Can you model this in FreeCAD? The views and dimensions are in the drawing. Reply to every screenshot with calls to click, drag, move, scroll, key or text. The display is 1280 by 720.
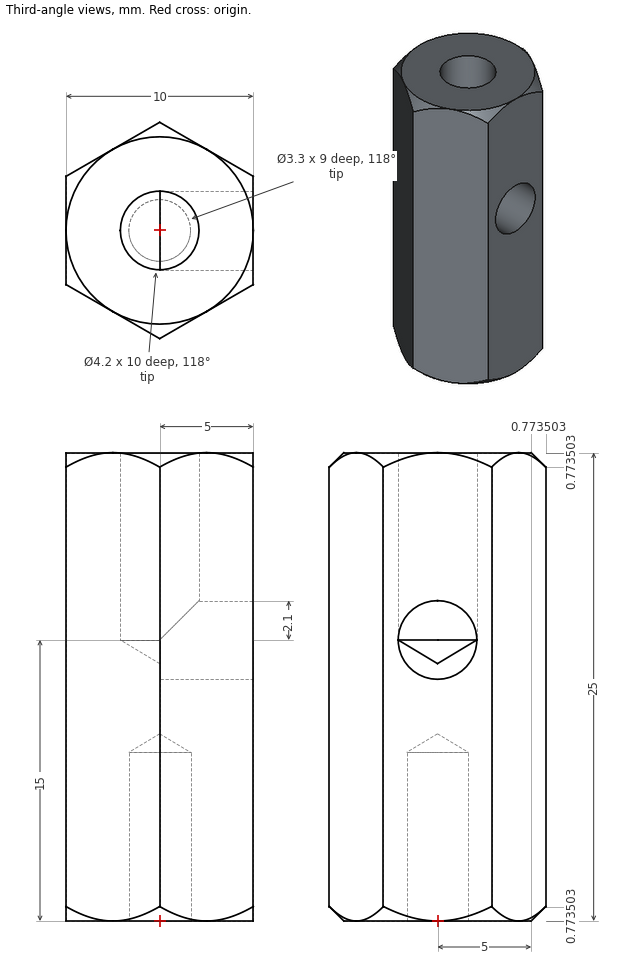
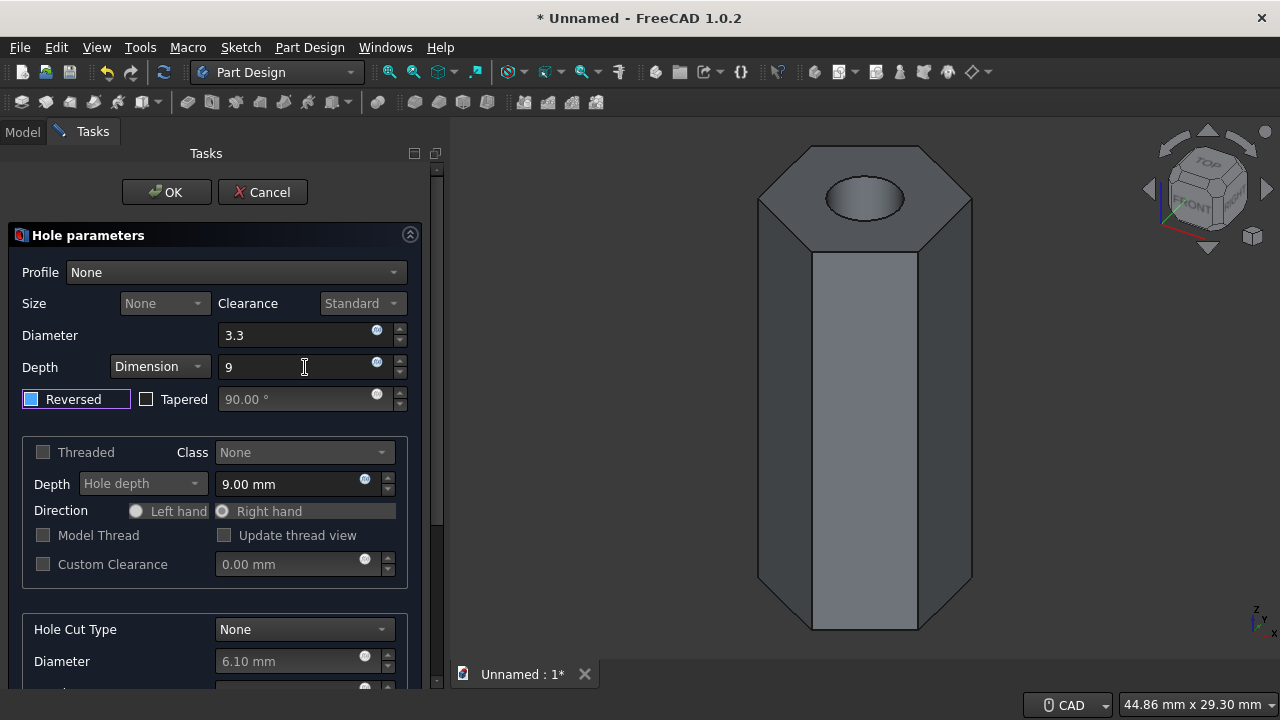
click(30, 399)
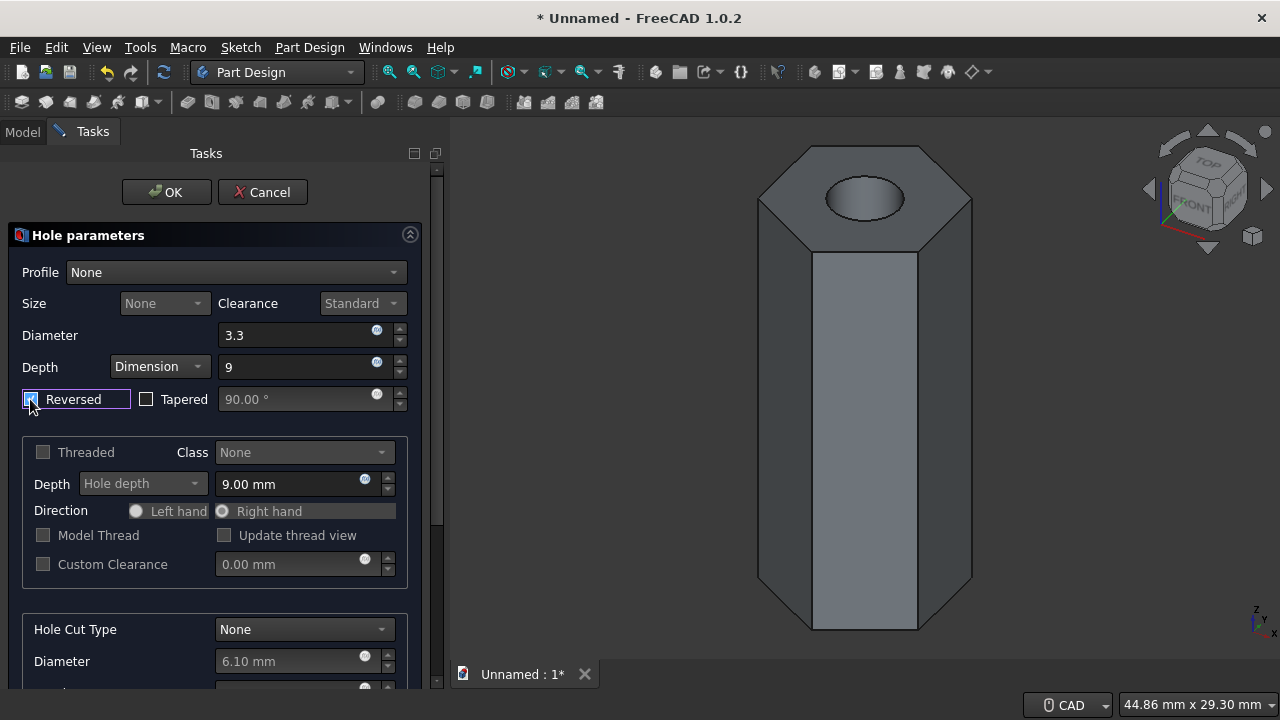
click(167, 192)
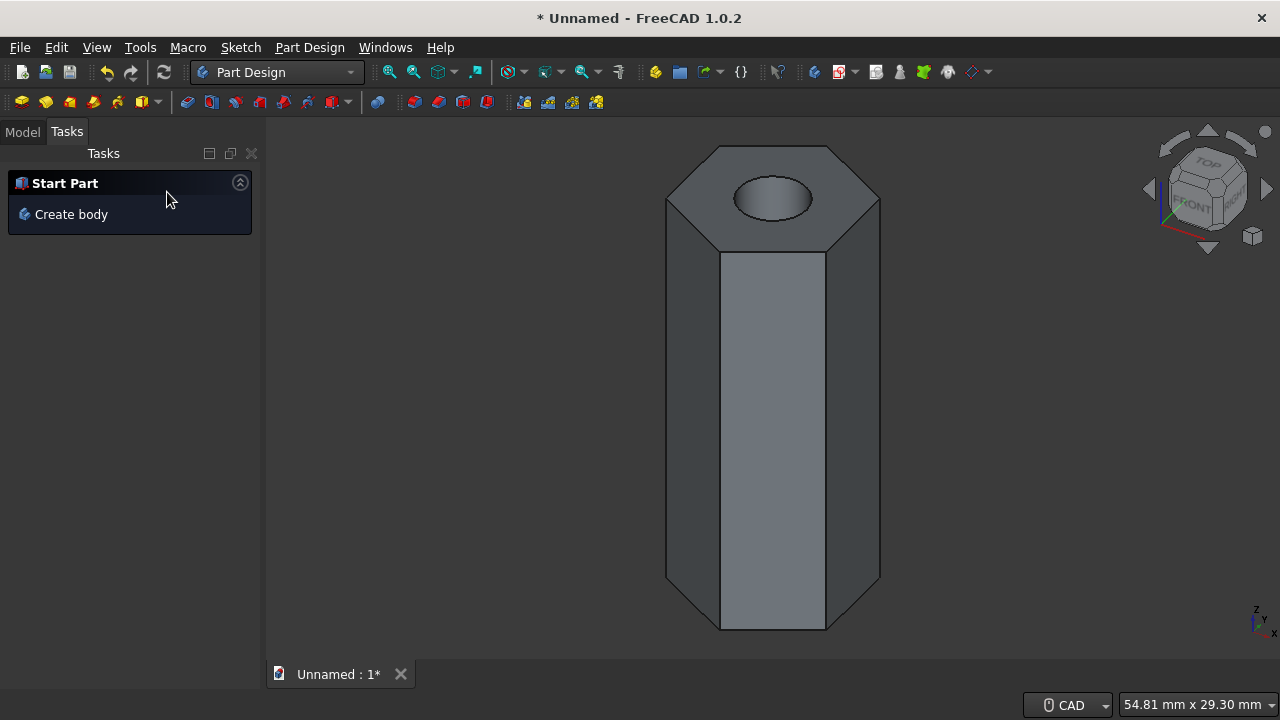
click(840, 72)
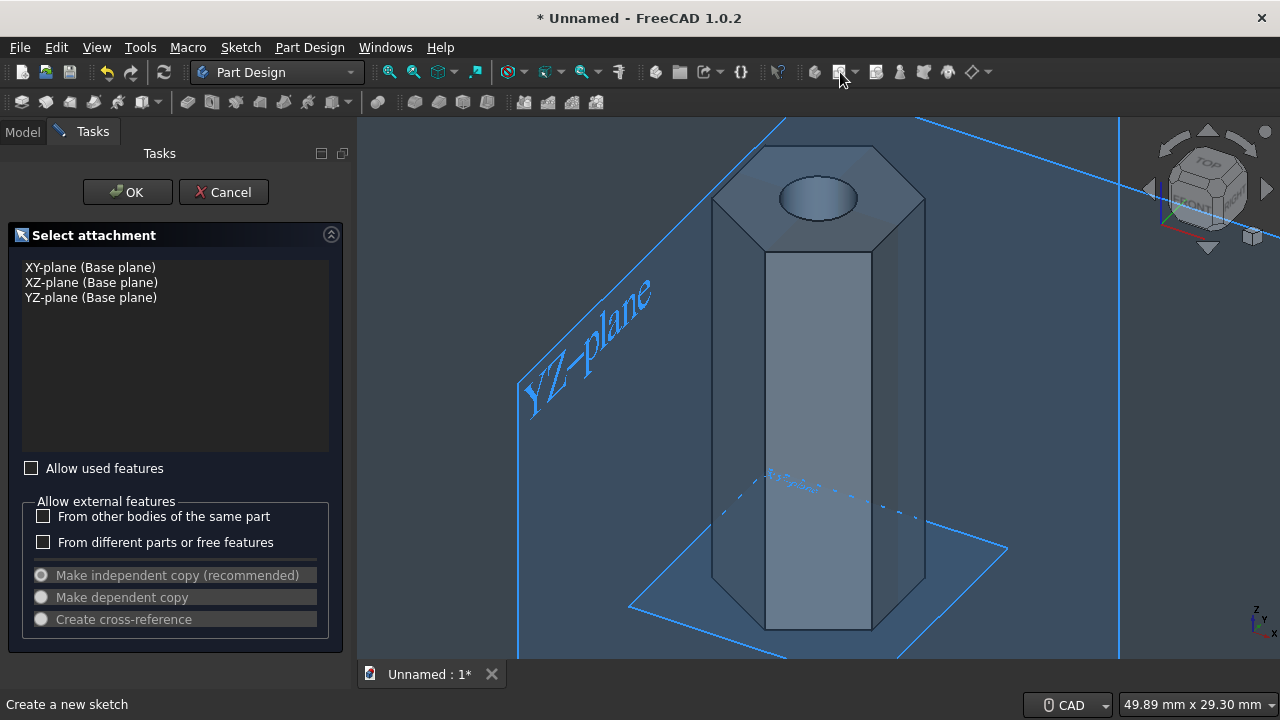
click(82, 282)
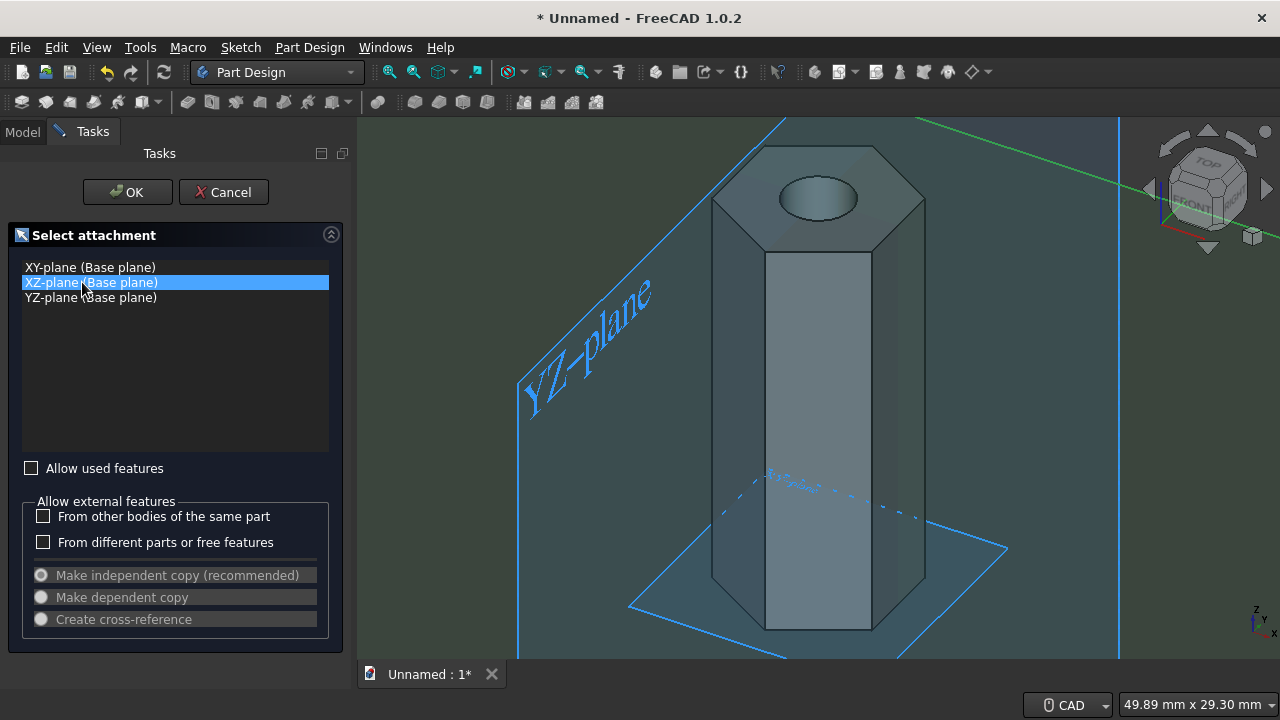
click(128, 192)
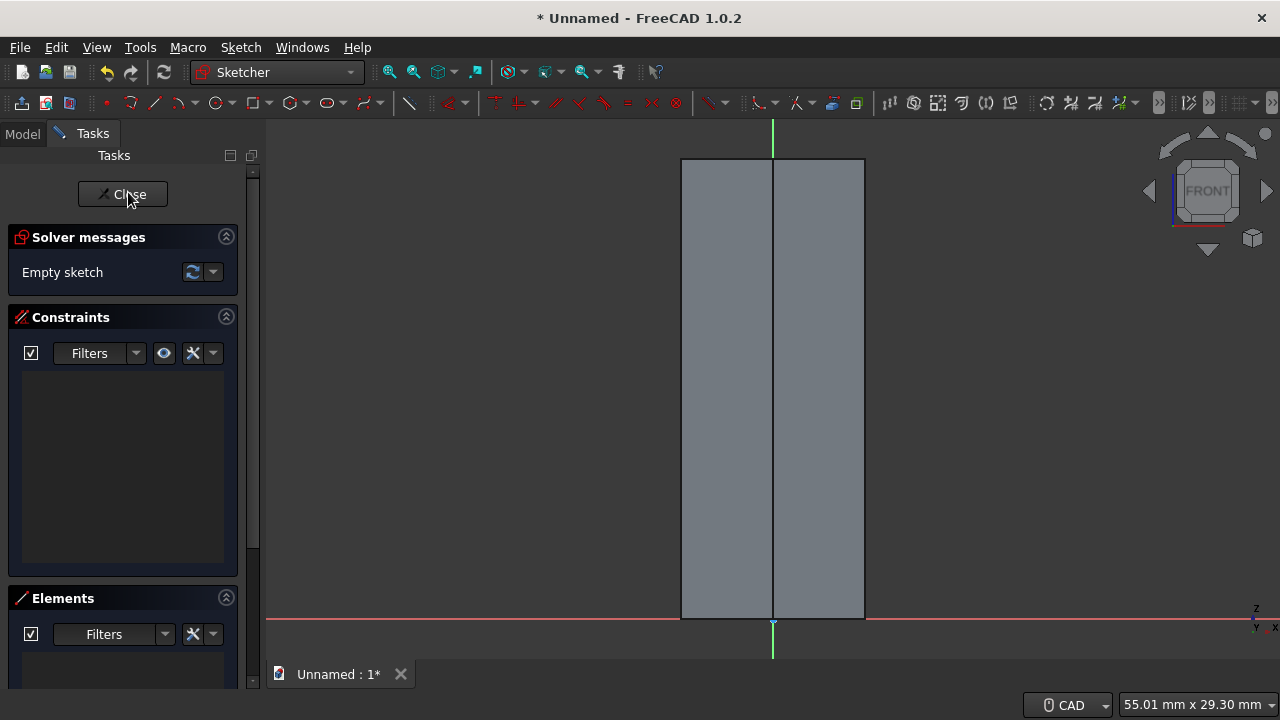
key(q)
key(s)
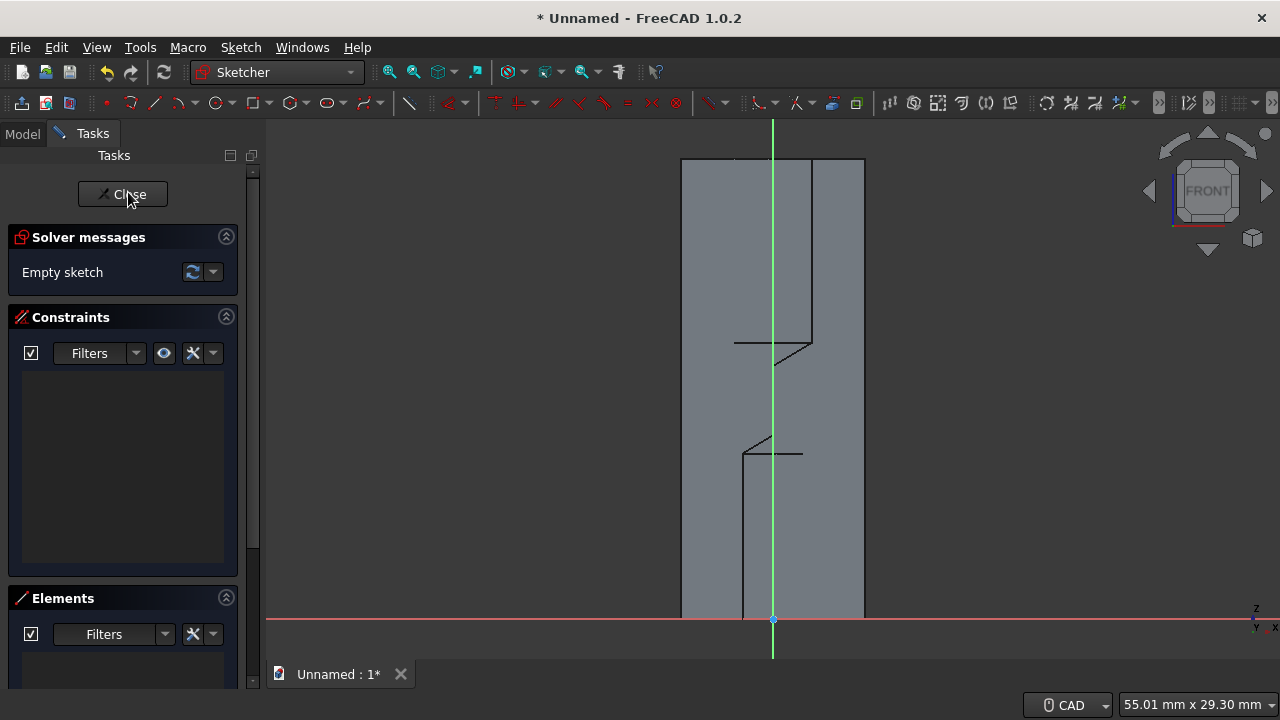
scroll(294, 147, down, 1)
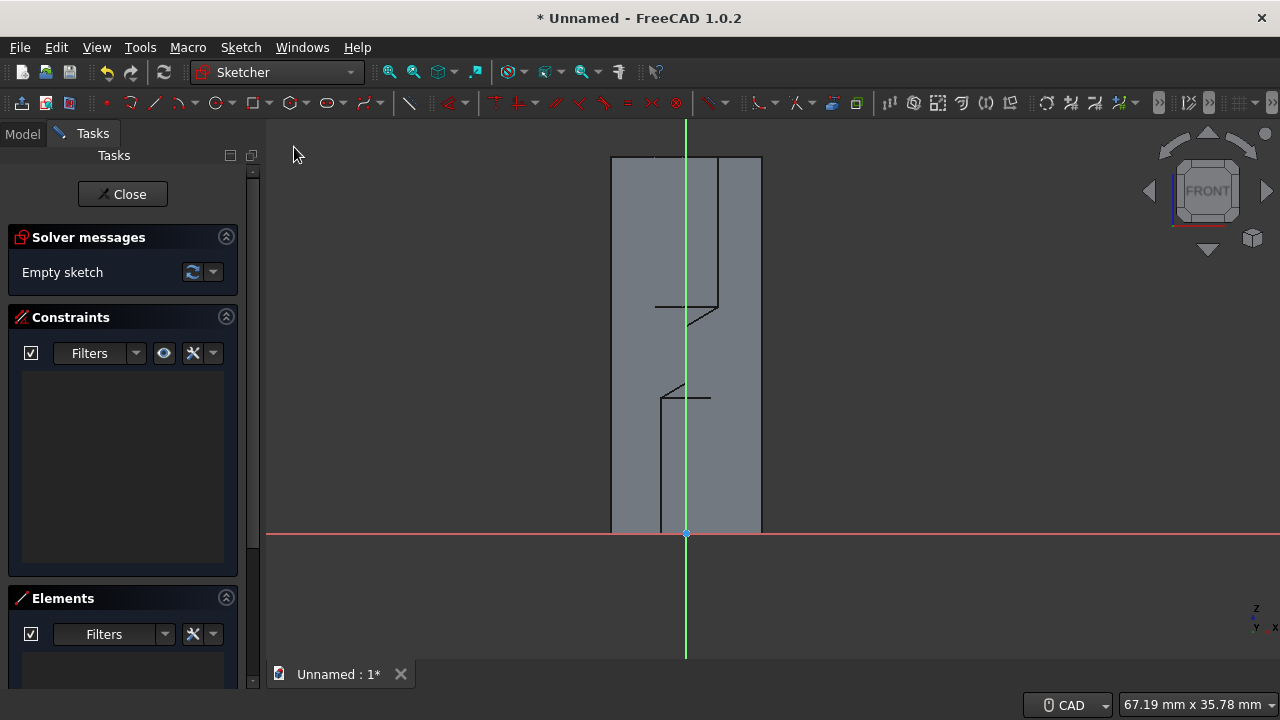
key(g)
key(r)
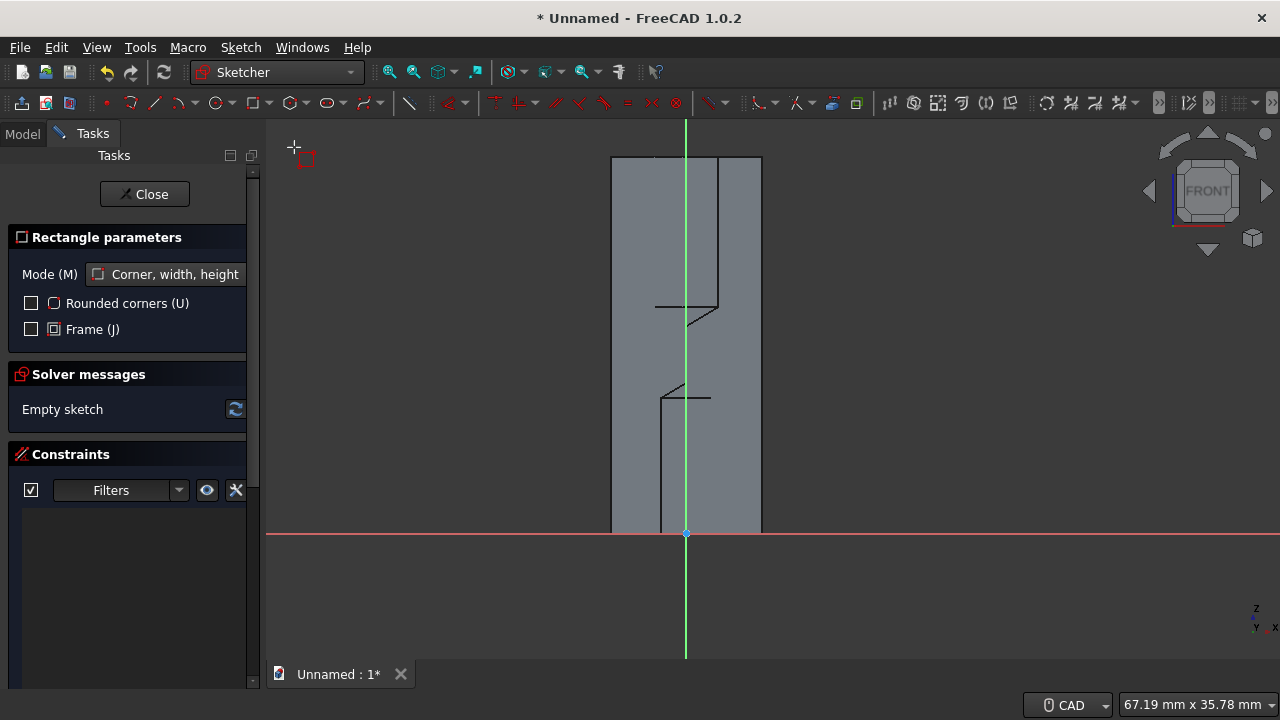
click(686, 276)
move(762, 307)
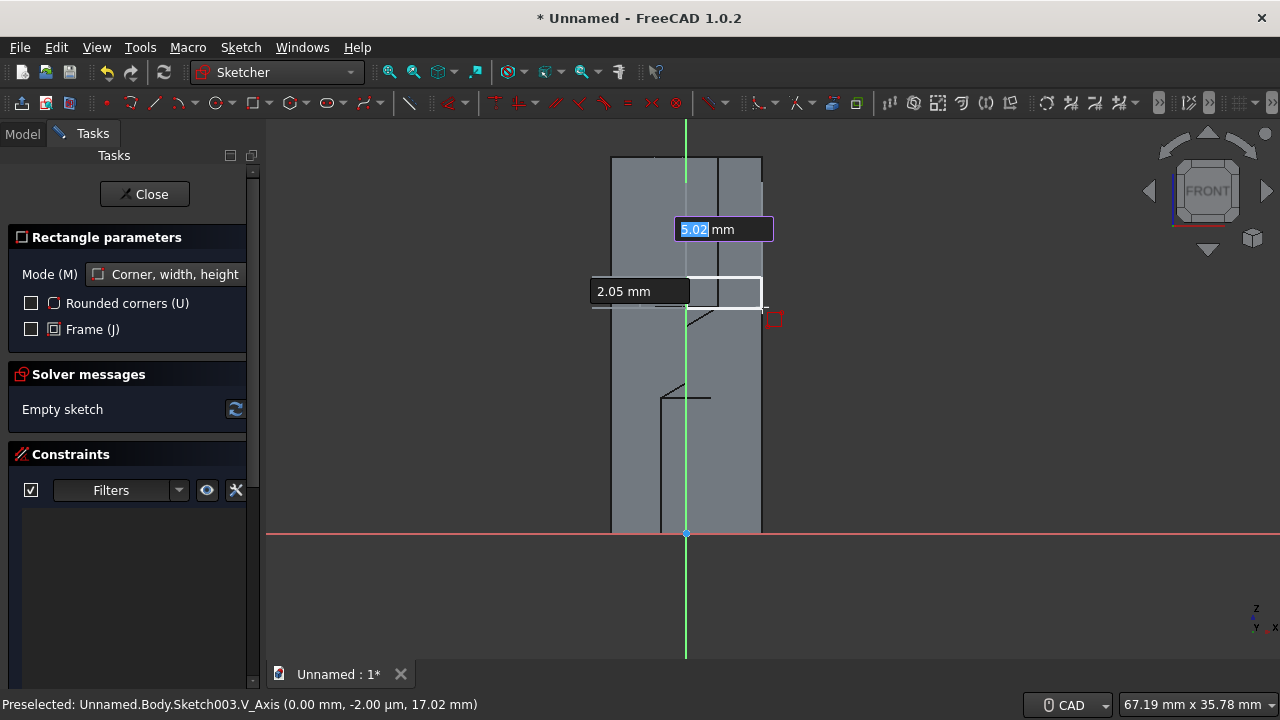
text(5)
key(Tab)
text(2.1)
key(Return)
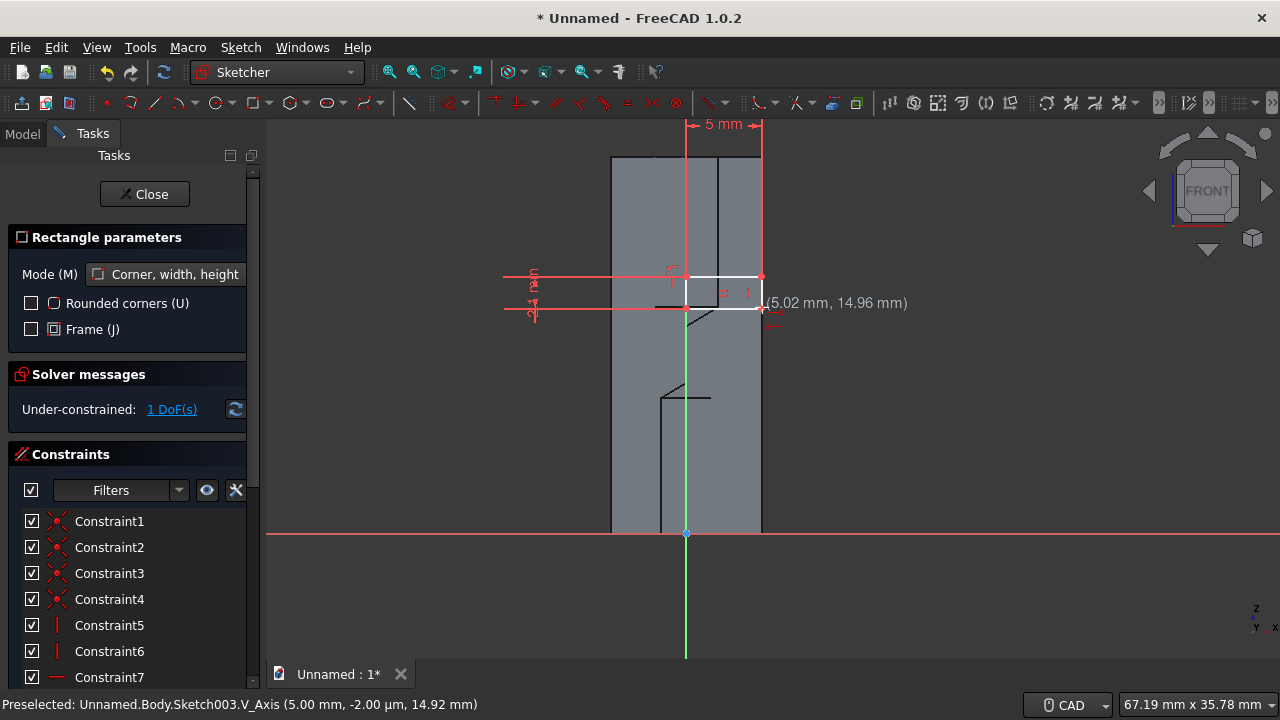
click(156, 104)